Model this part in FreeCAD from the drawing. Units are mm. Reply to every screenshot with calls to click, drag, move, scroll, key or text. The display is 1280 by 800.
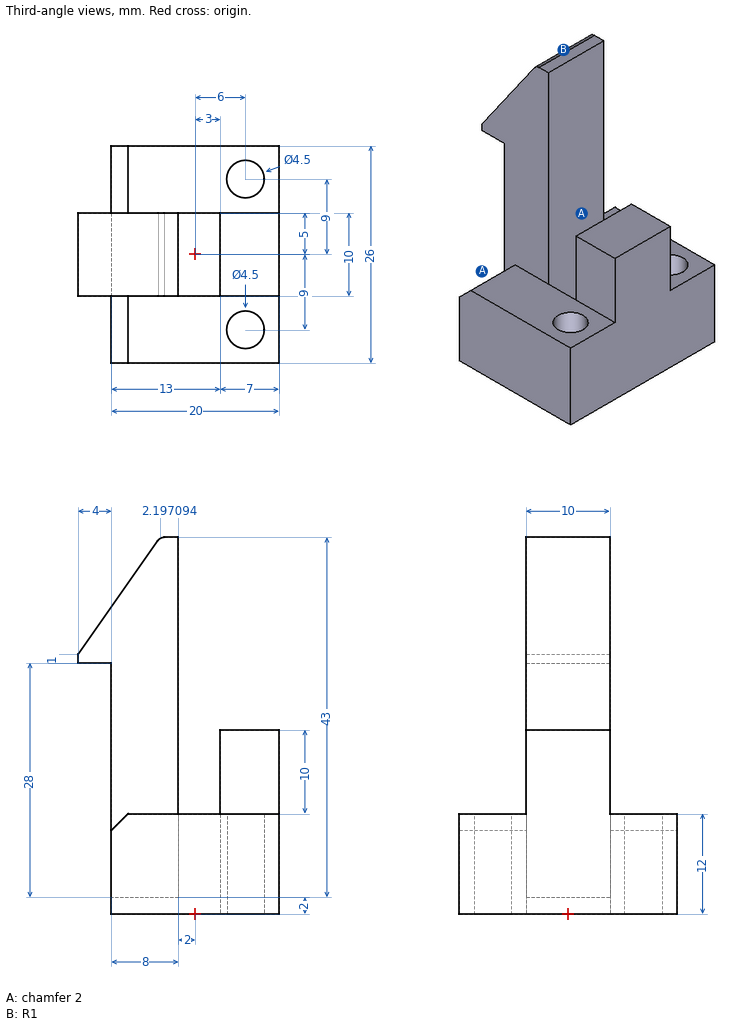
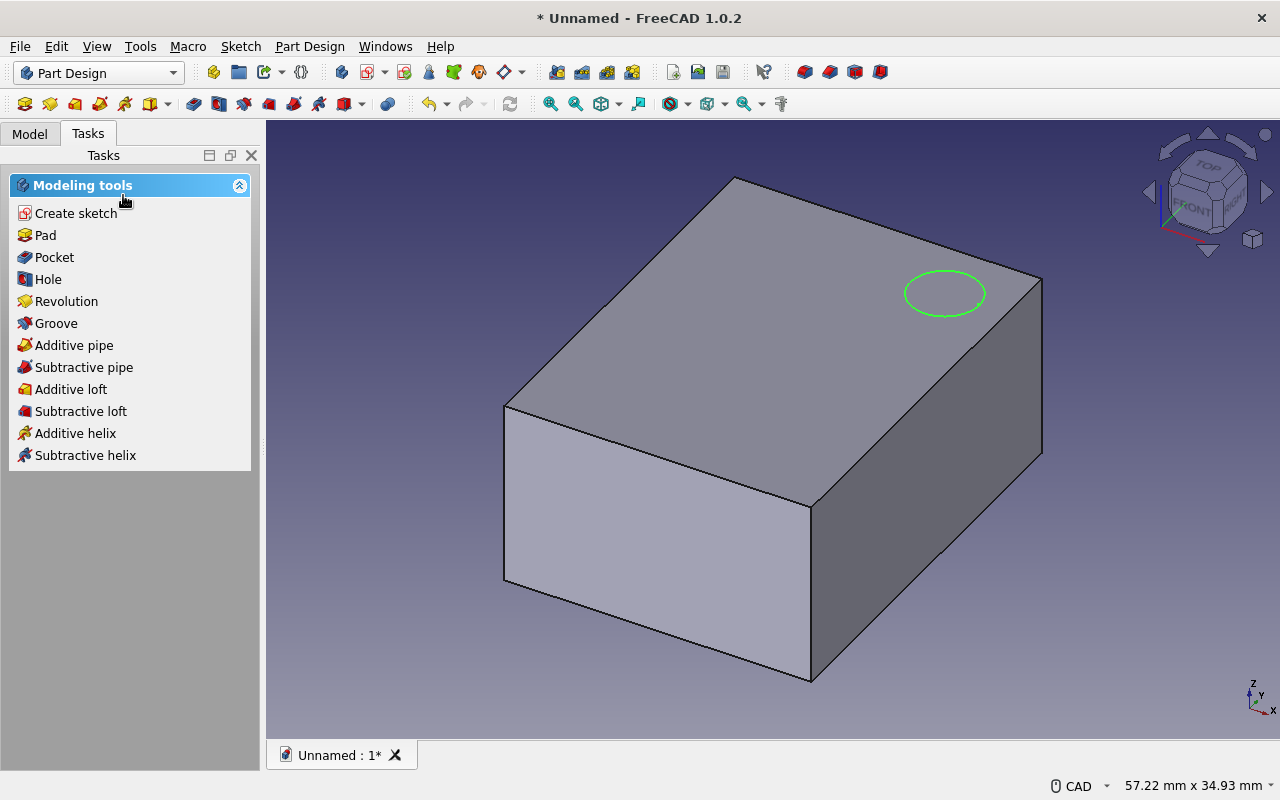
click(194, 104)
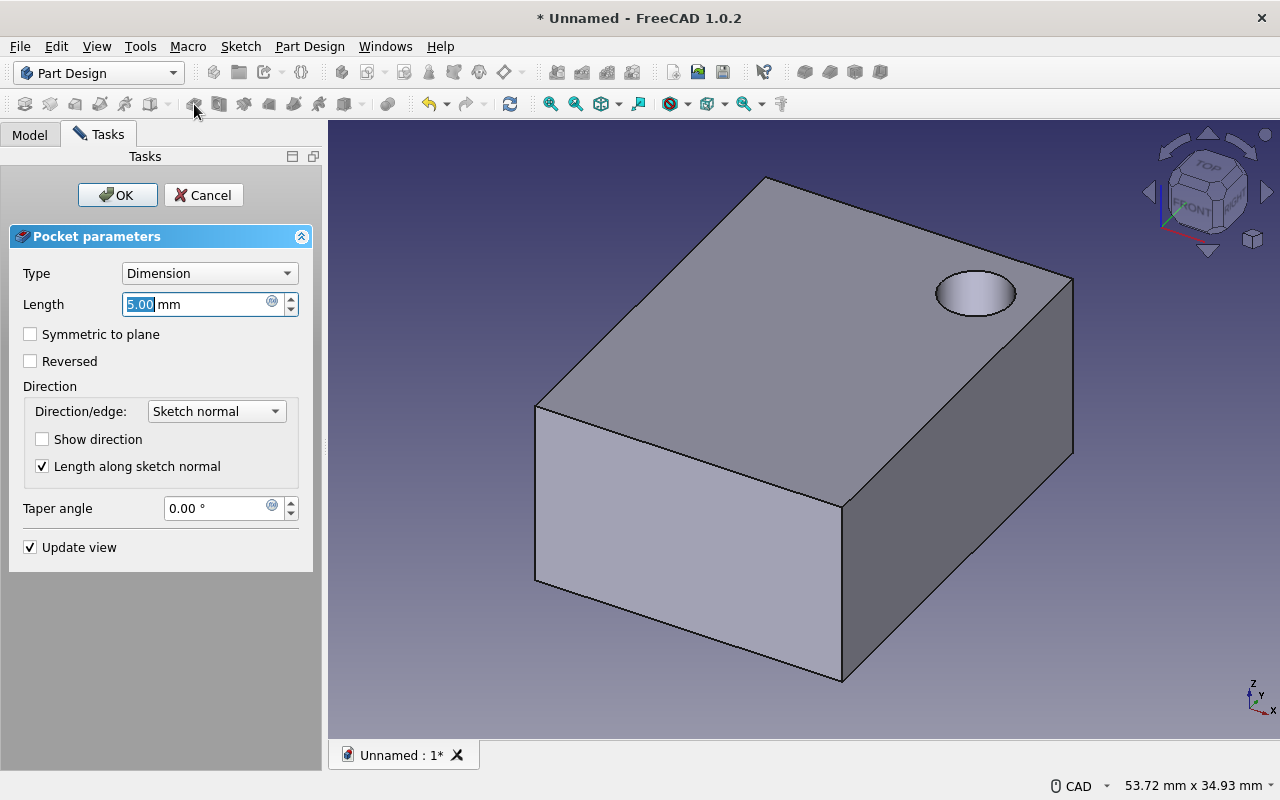
click(210, 274)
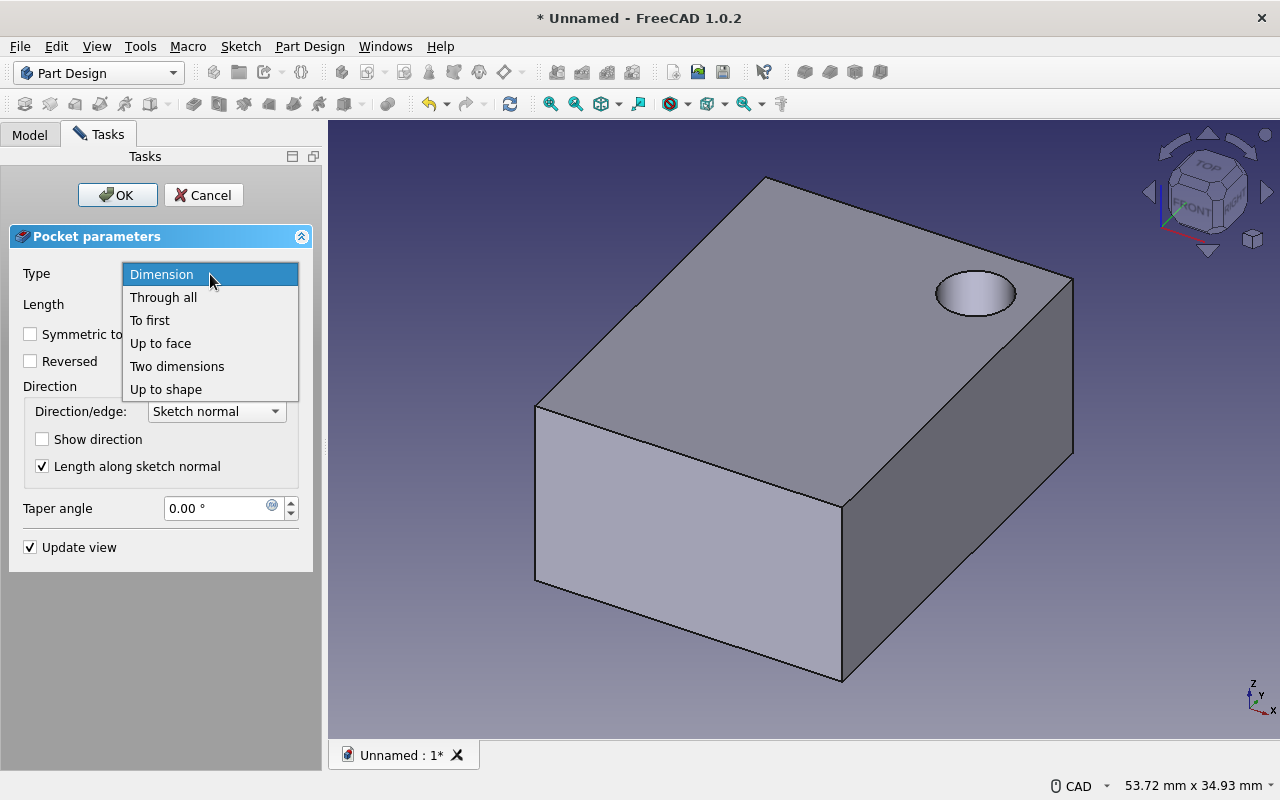
click(208, 320)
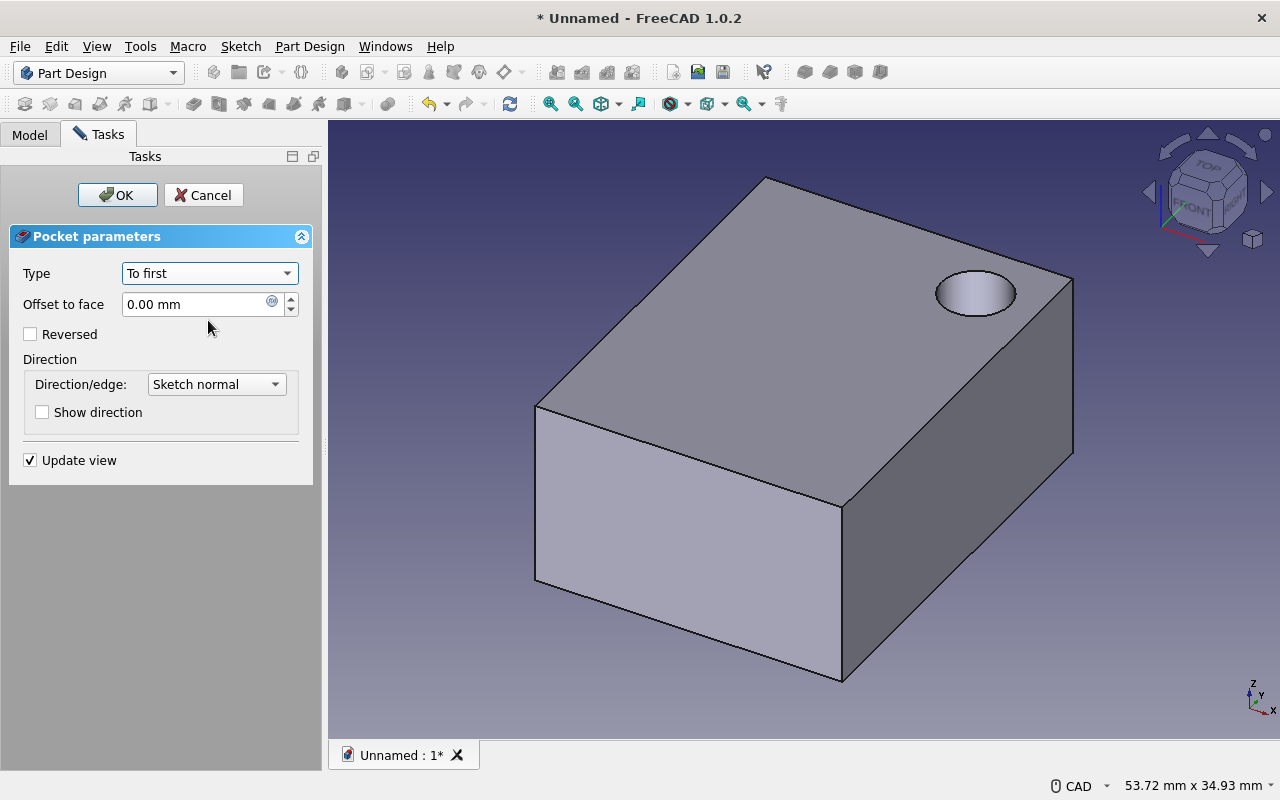
click(118, 195)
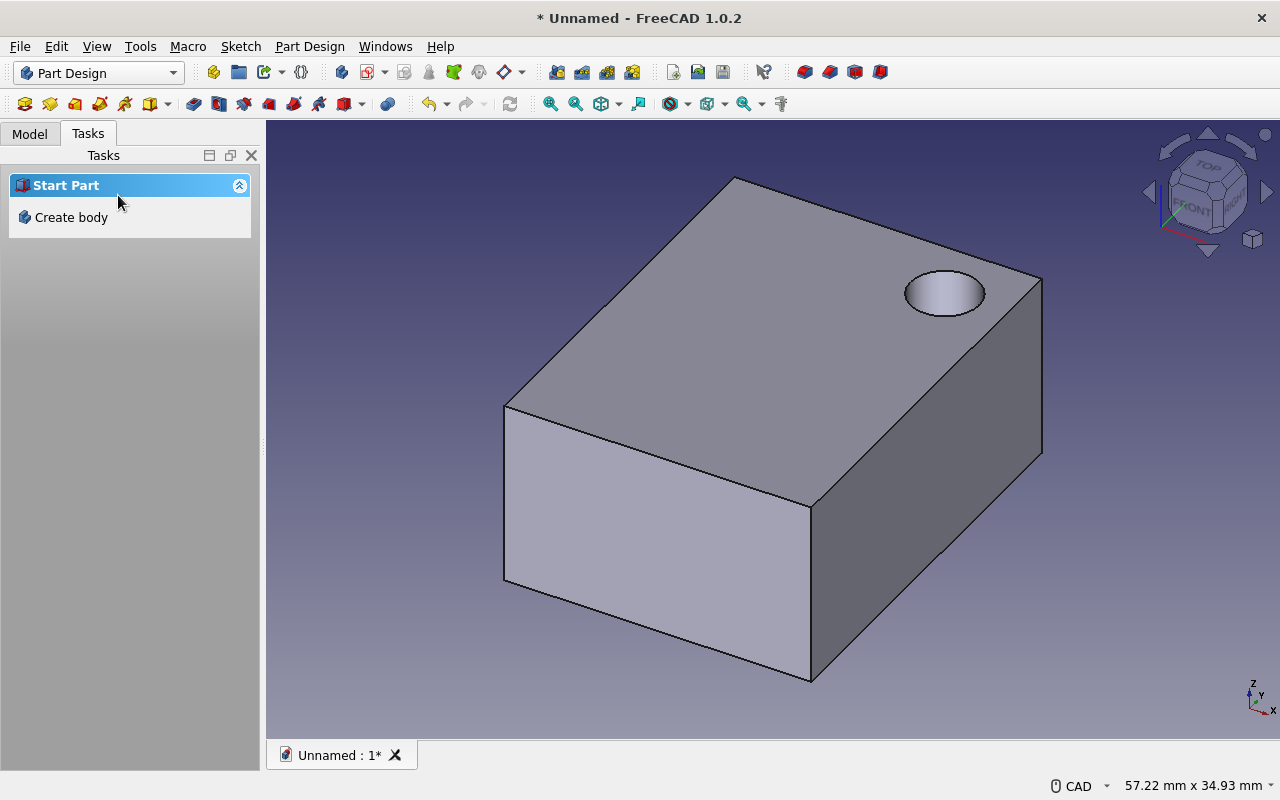
click(740, 374)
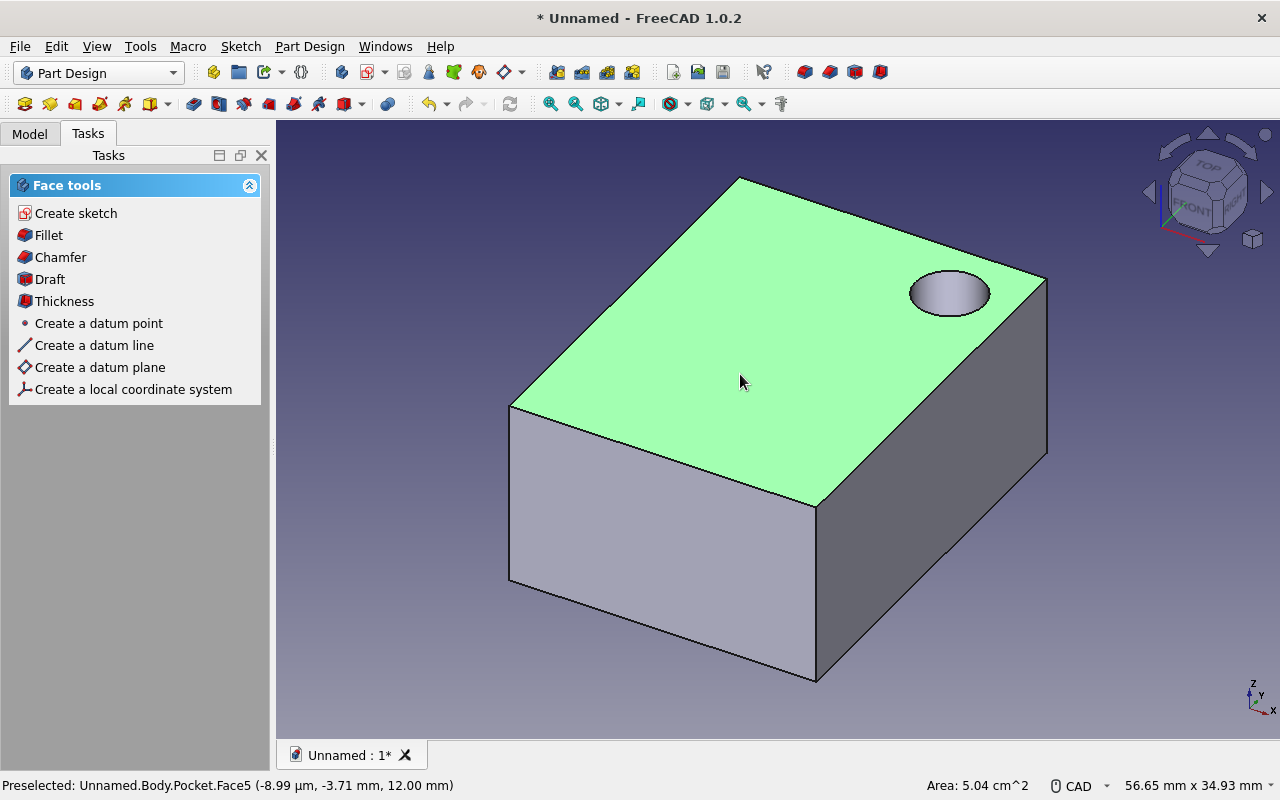
click(366, 72)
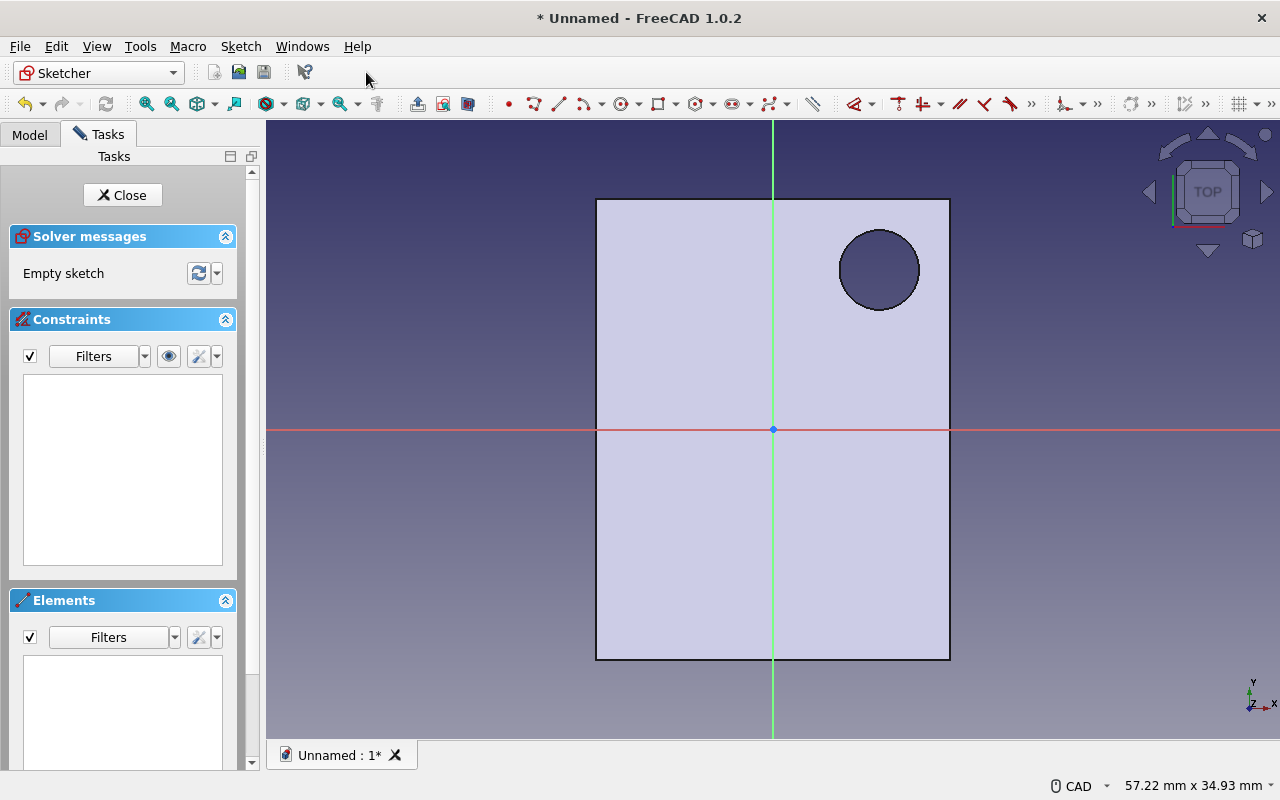
scroll(924, 629, up, 8)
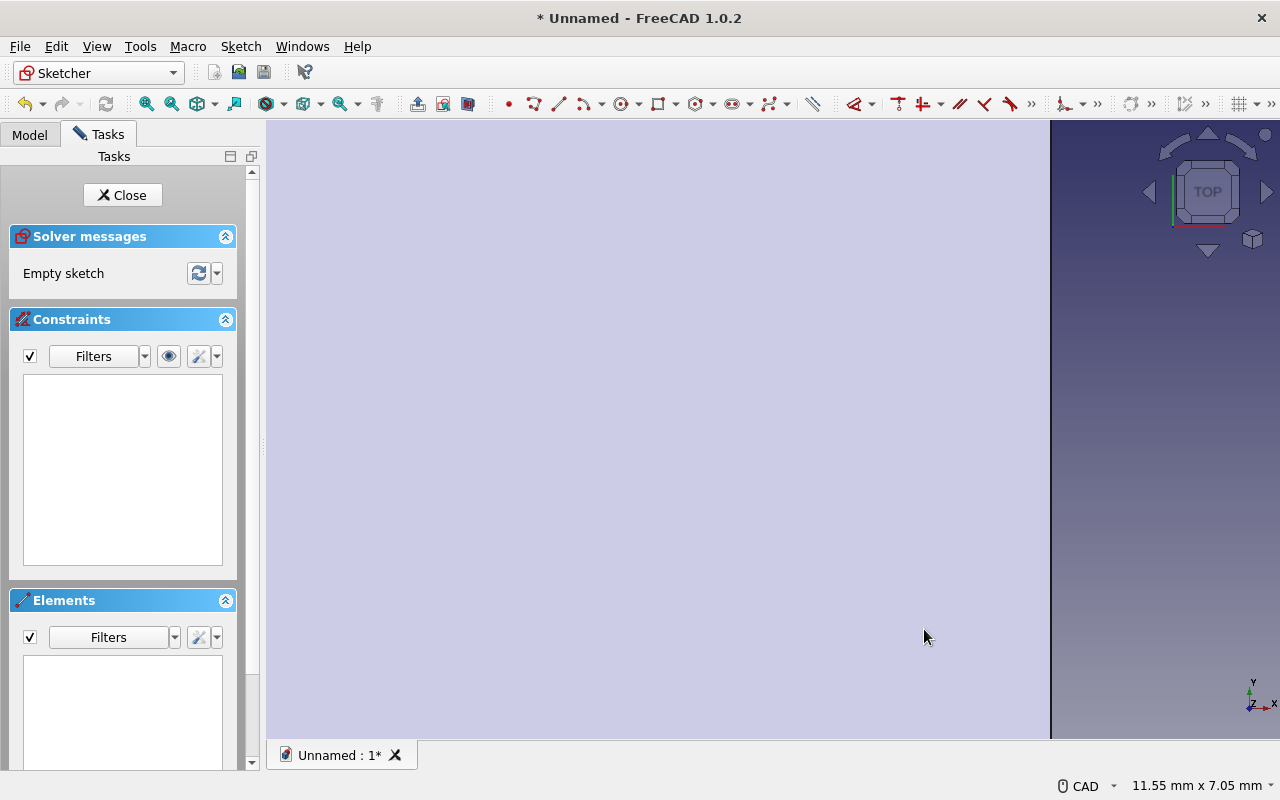
key(g)
key(c)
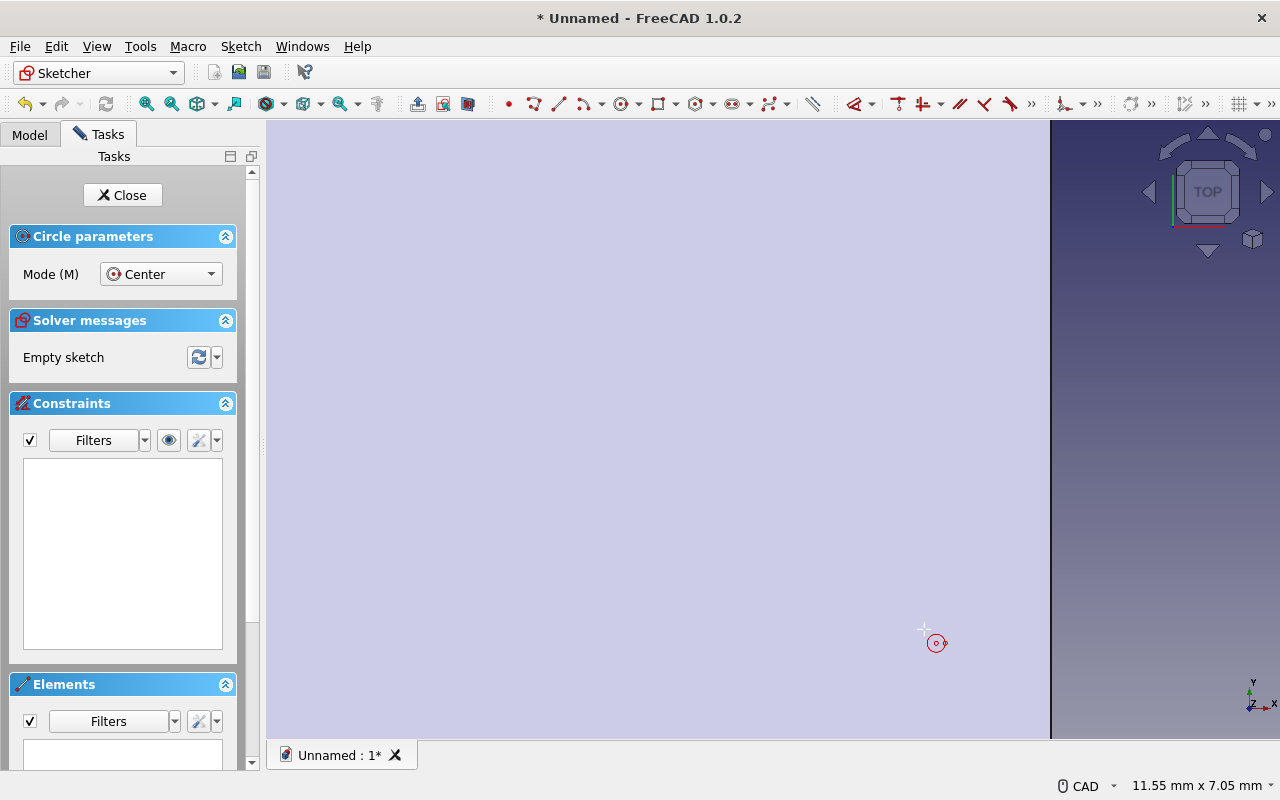
click(700, 428)
click(840, 288)
key(Escape)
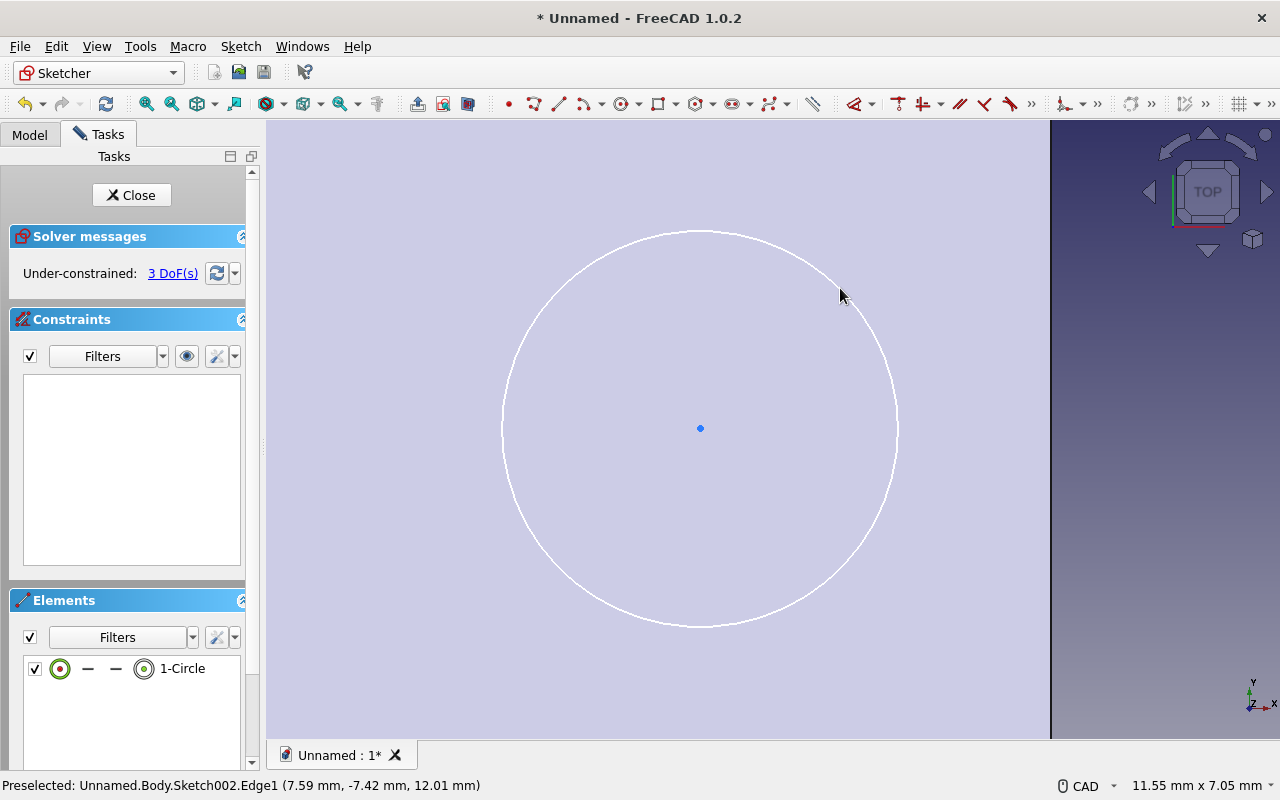
key(d)